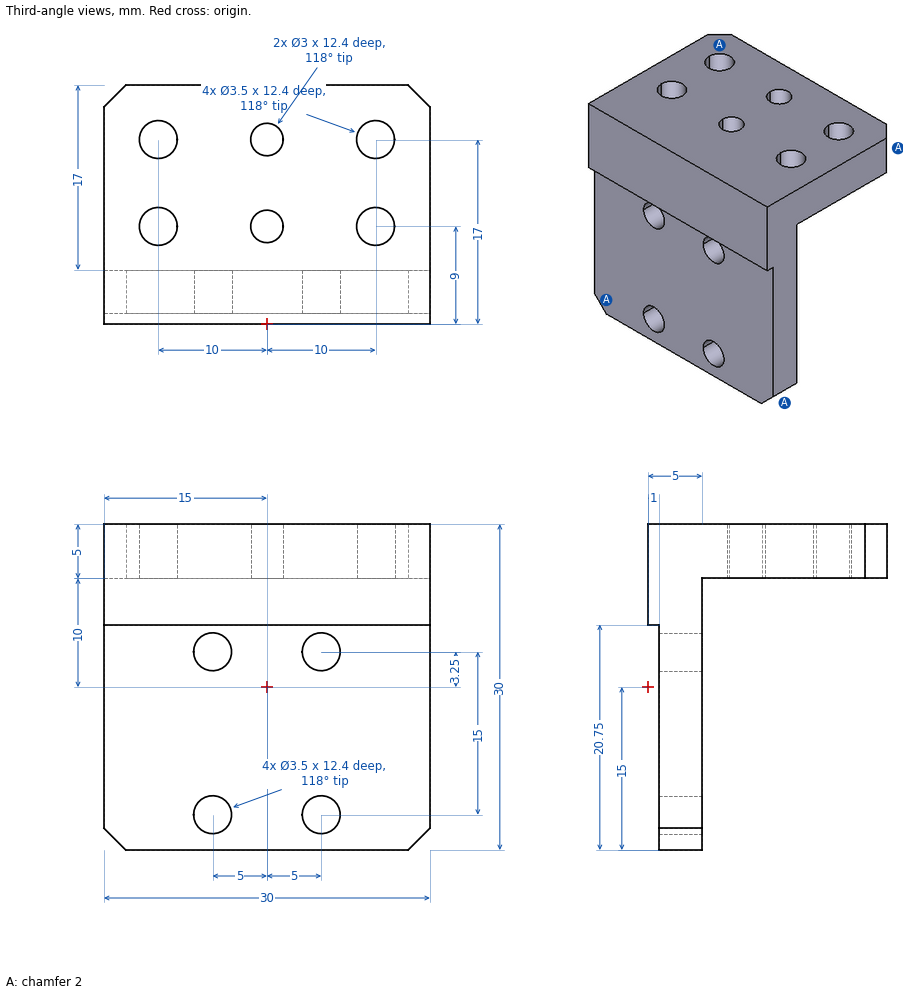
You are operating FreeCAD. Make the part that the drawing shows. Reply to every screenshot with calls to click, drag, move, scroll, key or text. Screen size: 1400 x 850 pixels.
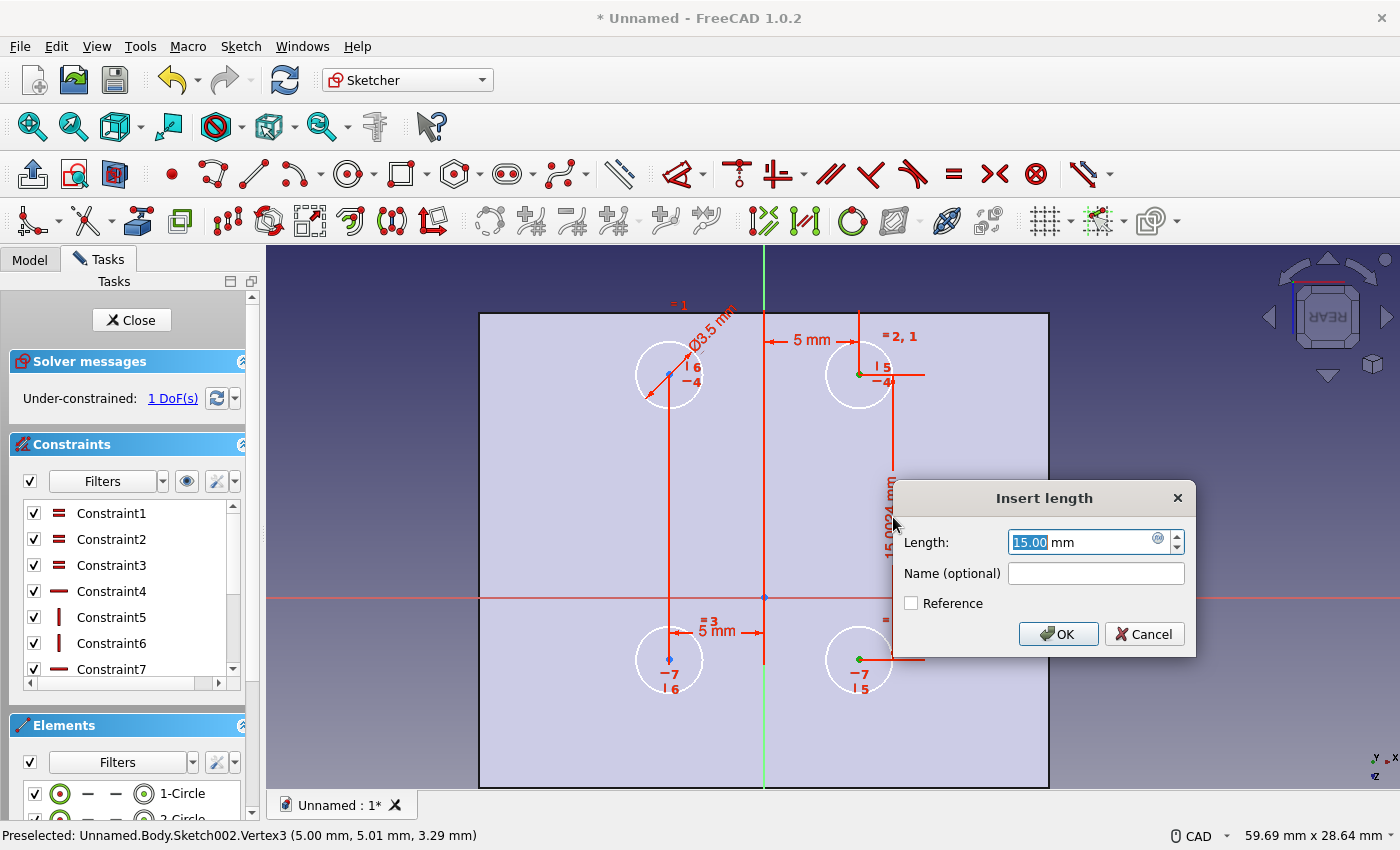
text(15)
key(Return)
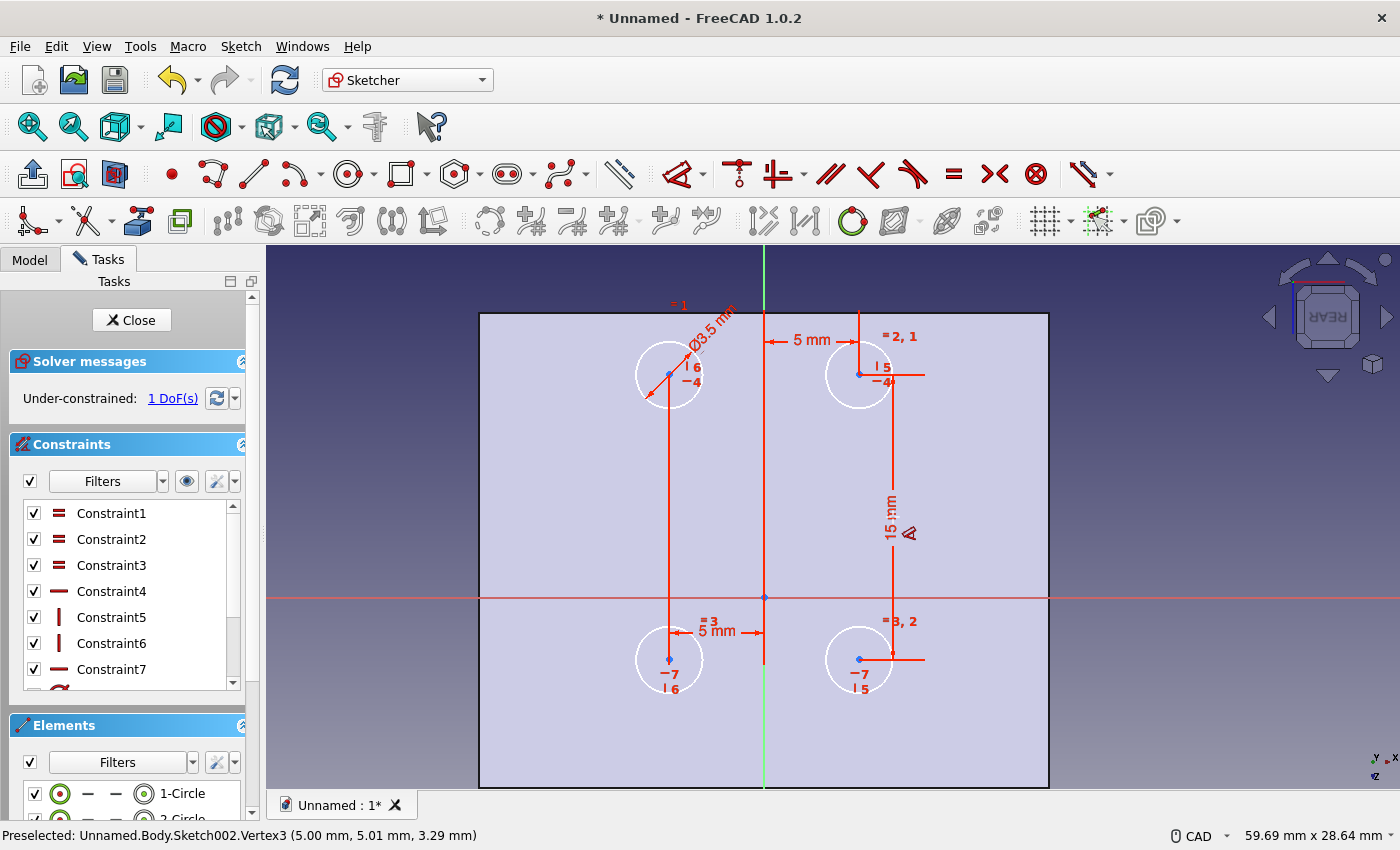
click(859, 660)
click(893, 614)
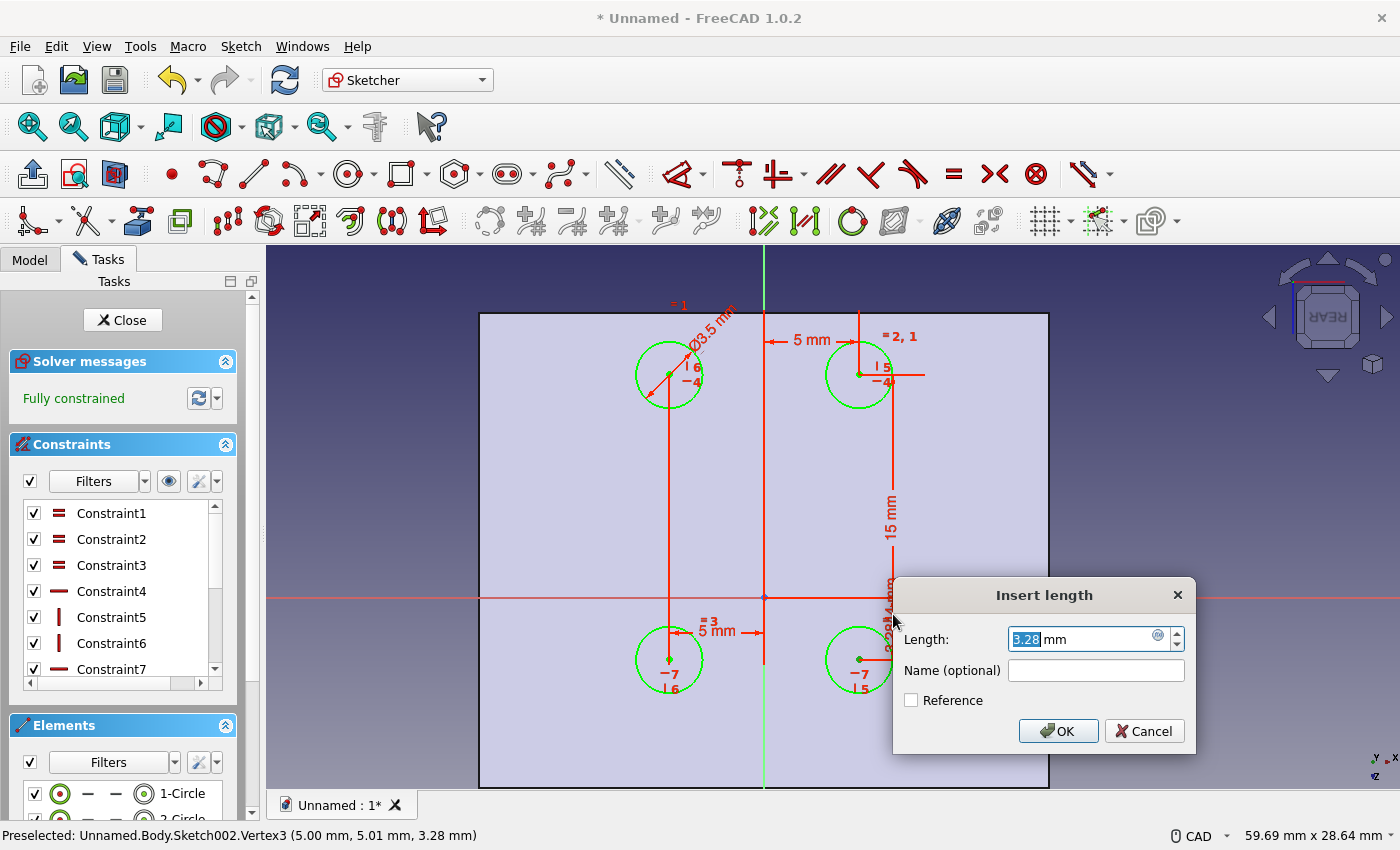
text(3.25)
key(Return)
key(Escape)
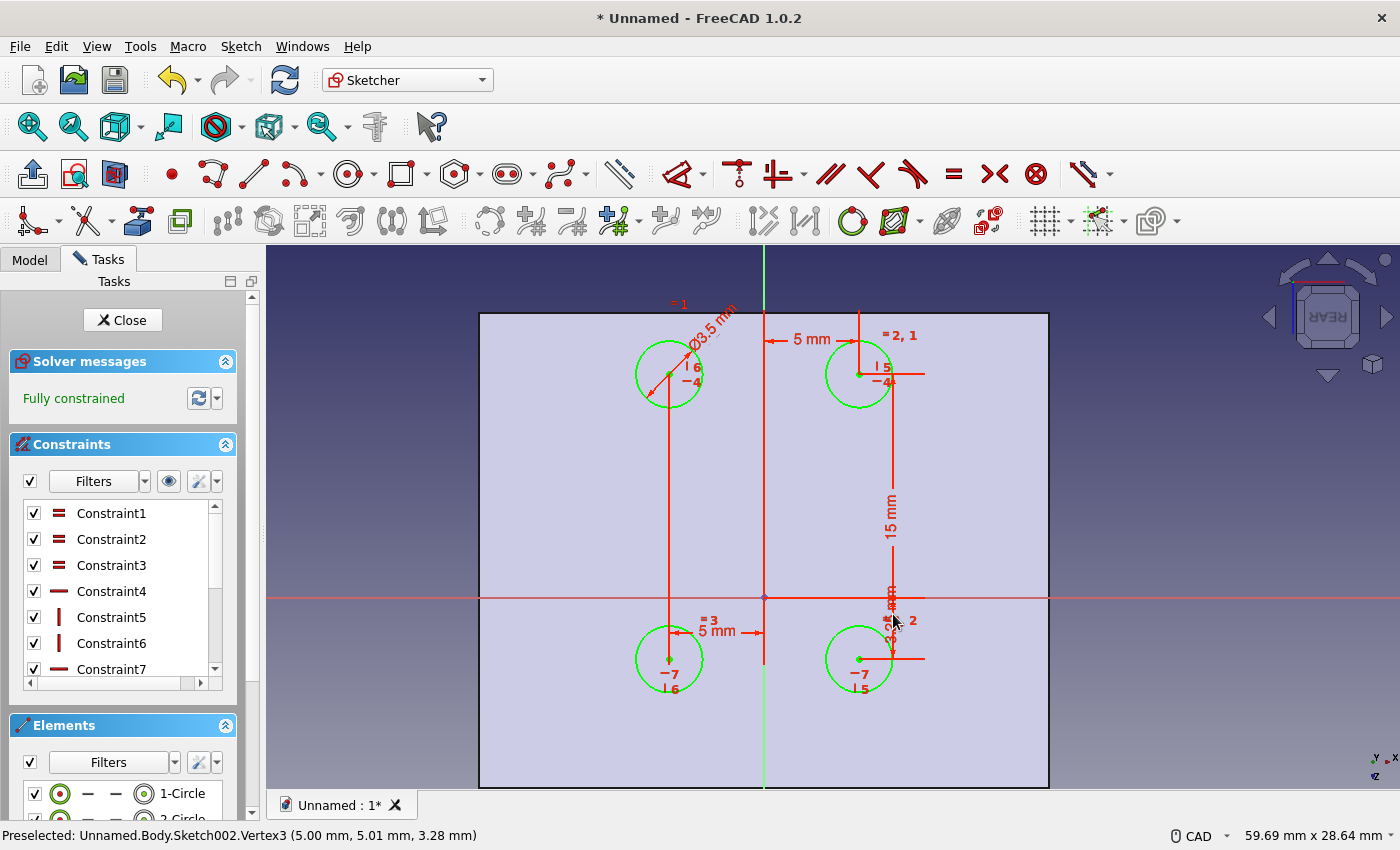
click(123, 320)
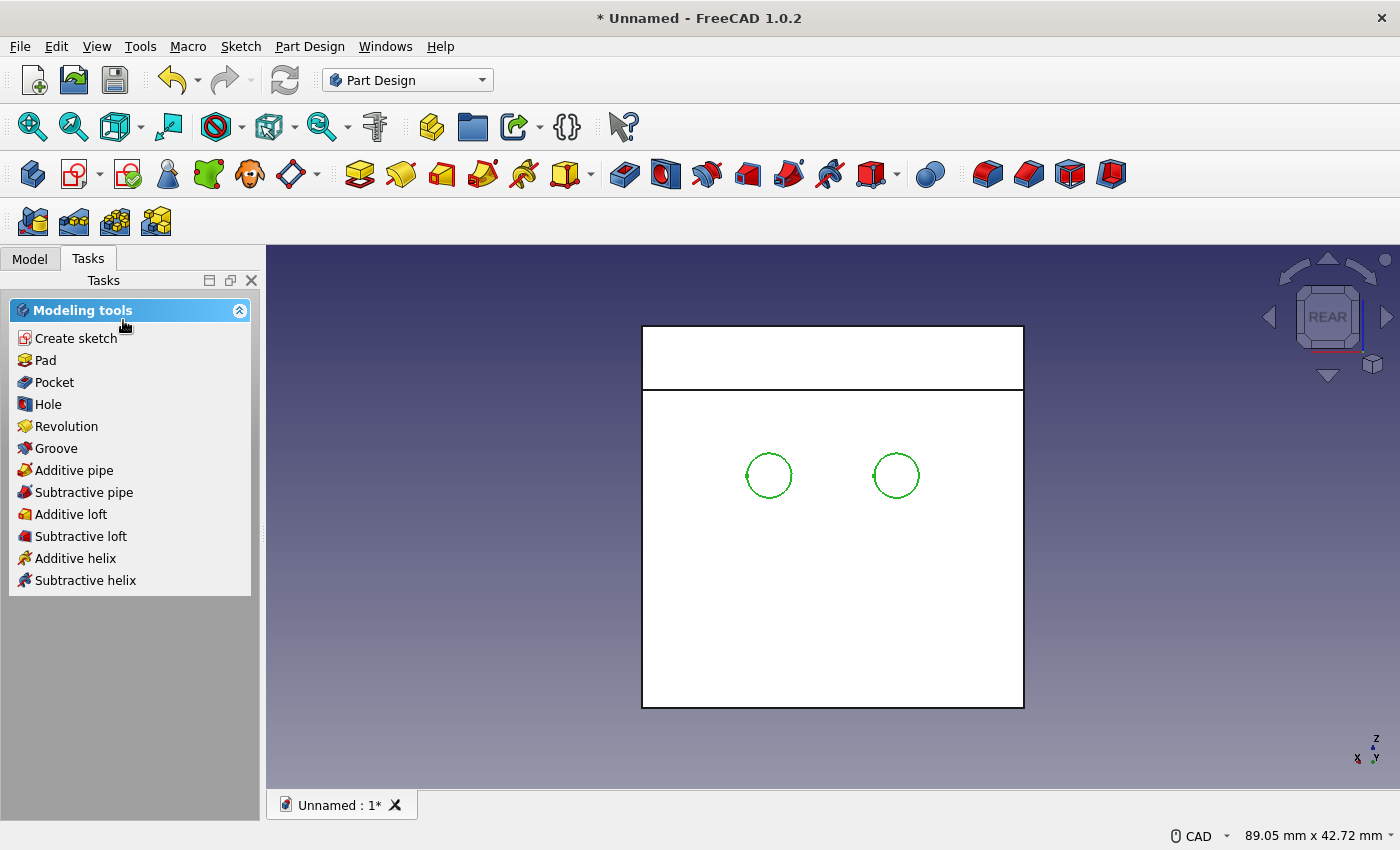
click(666, 174)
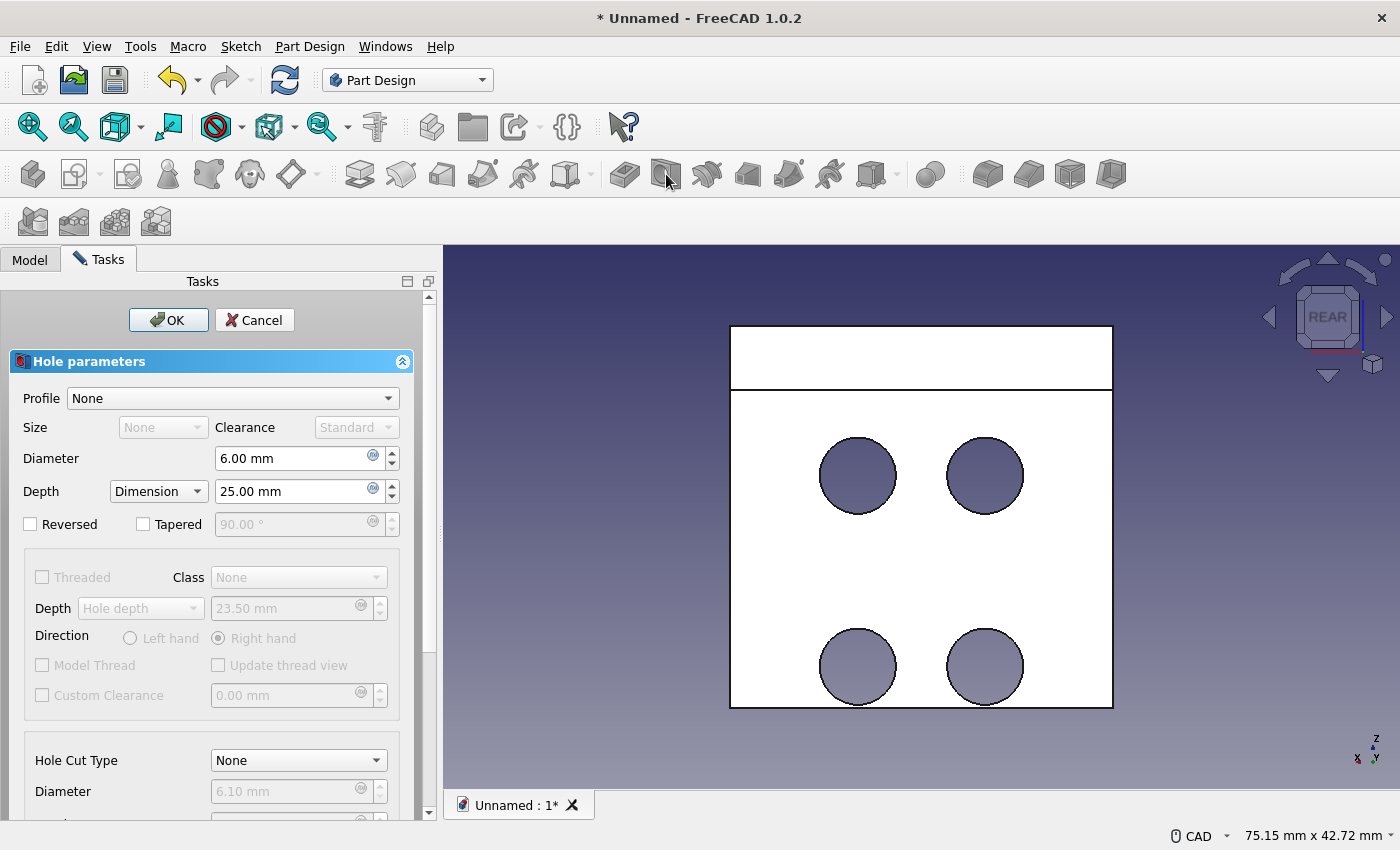
triple_click(300, 458)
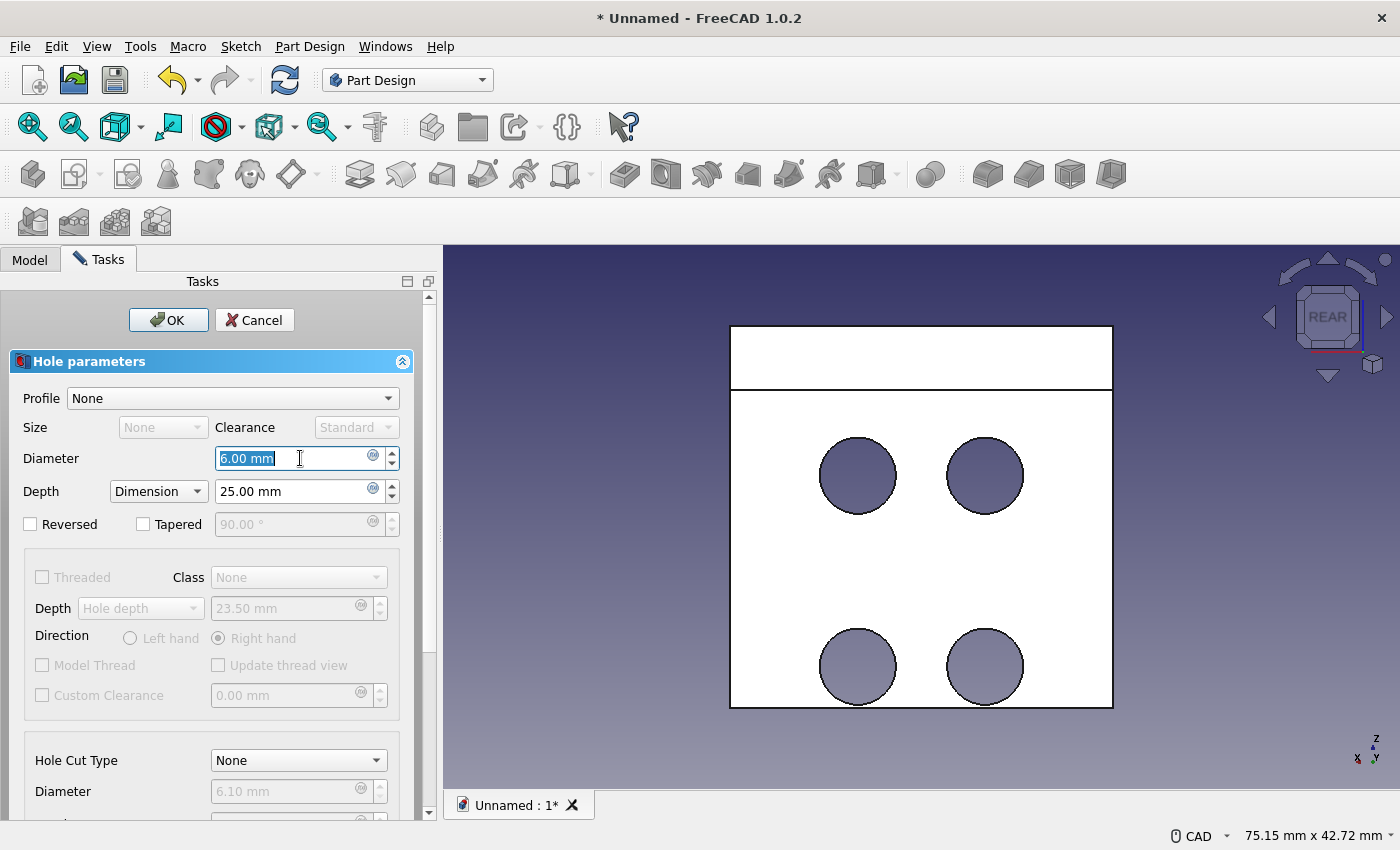
text(3.5)
key(Tab)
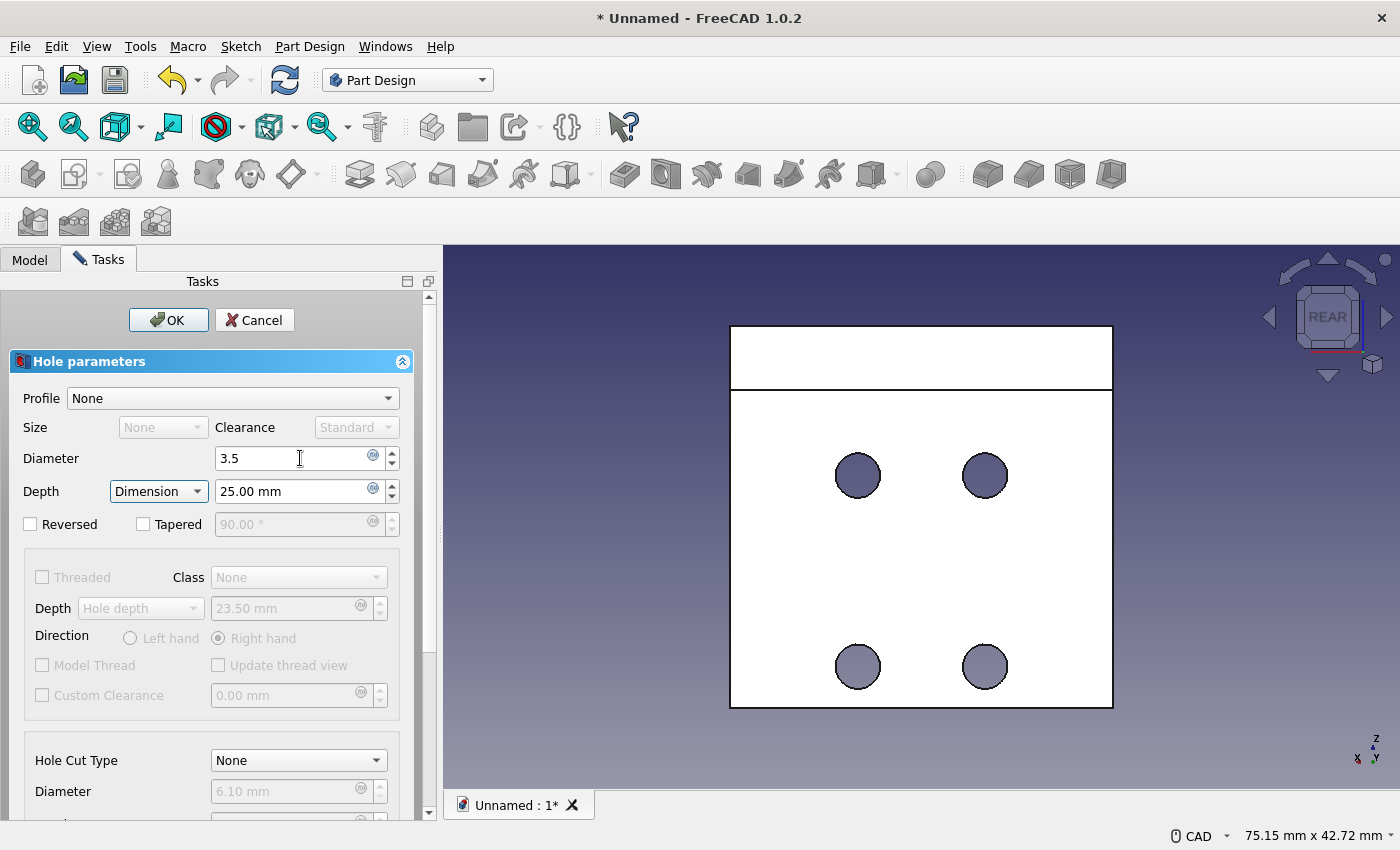
triple_click(300, 492)